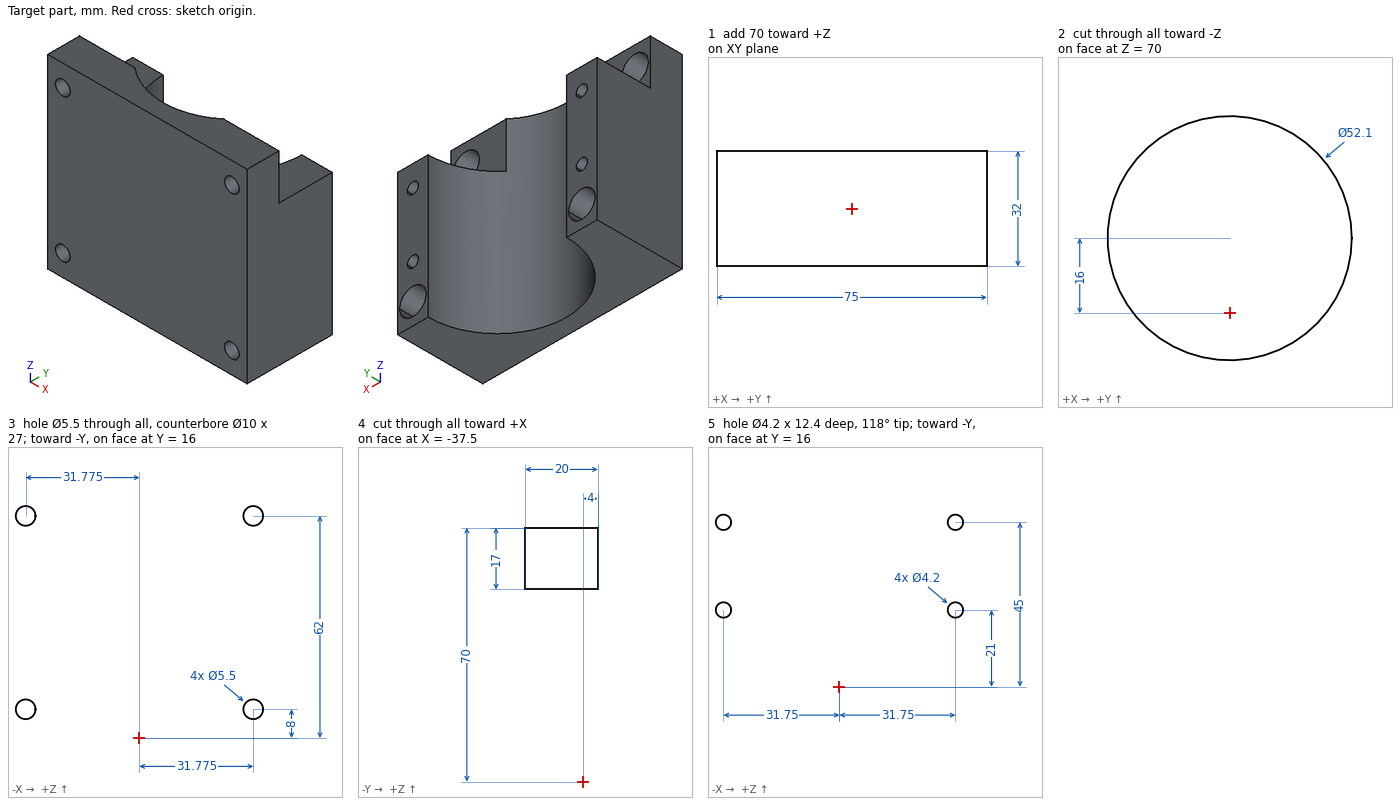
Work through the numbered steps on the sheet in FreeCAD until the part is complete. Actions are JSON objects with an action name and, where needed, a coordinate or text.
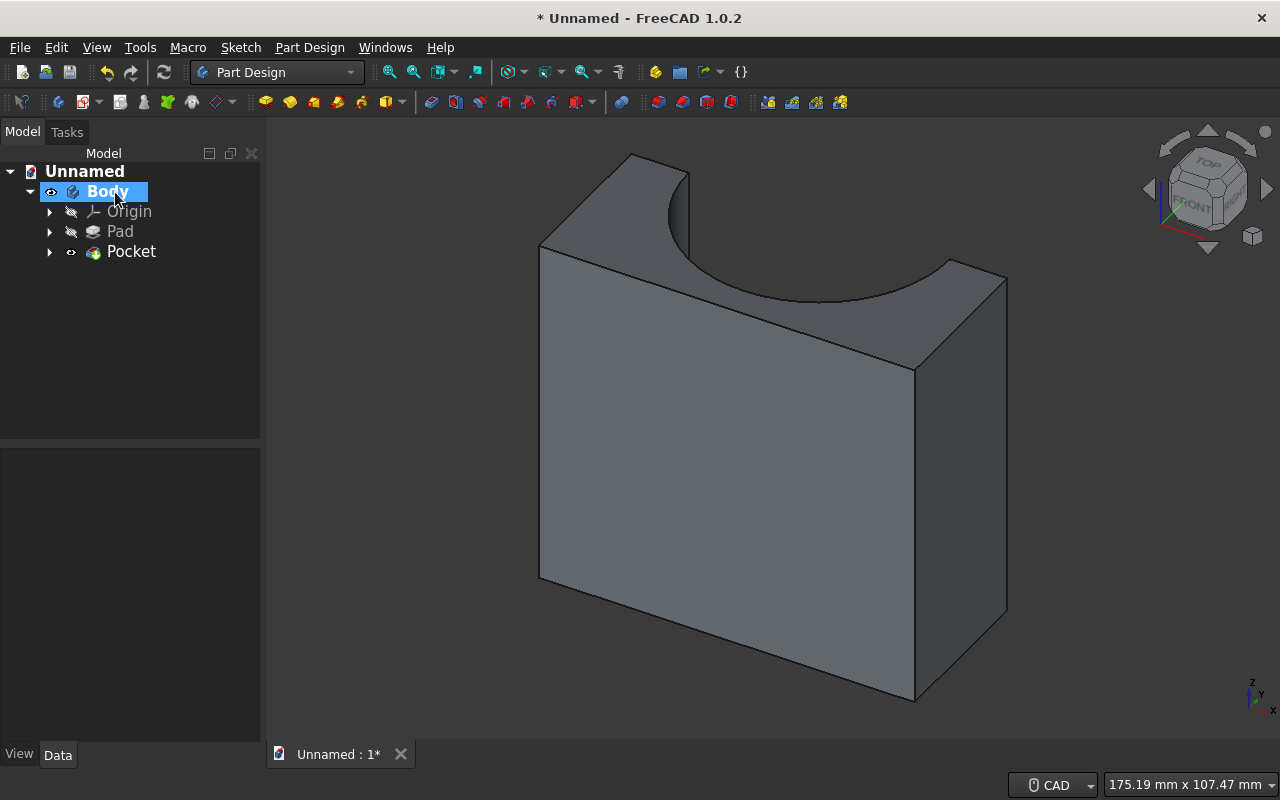
{"action": "key", "text": "4"}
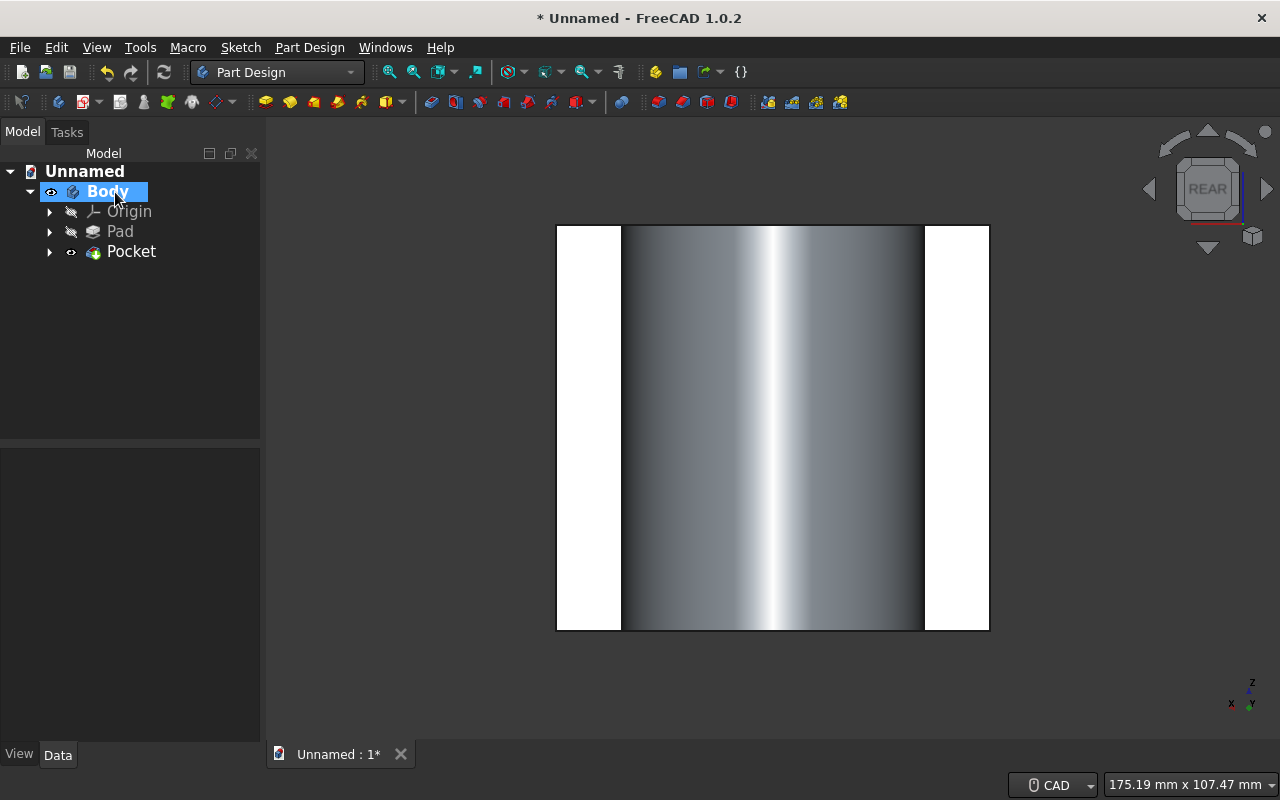
{"action": "left_click", "coordinate": [957, 311]}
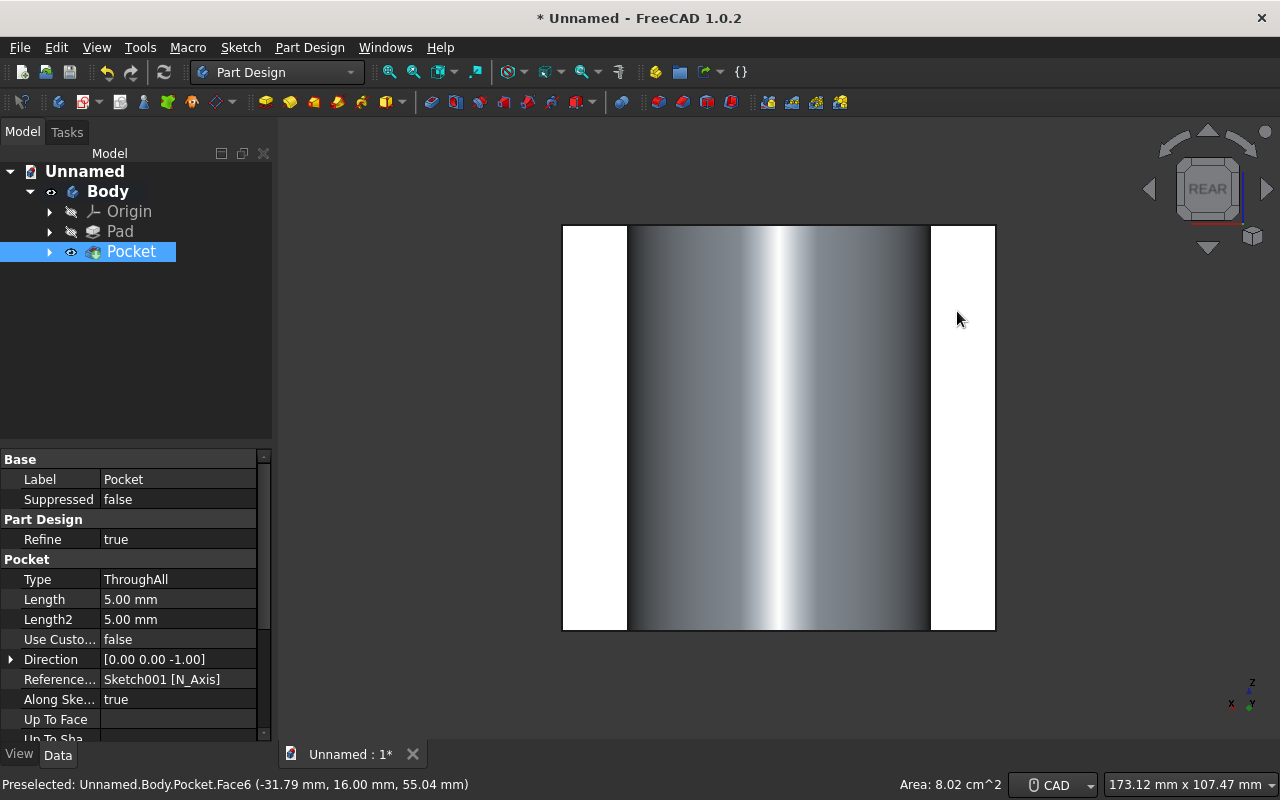
{"action": "left_click", "coordinate": [84, 102]}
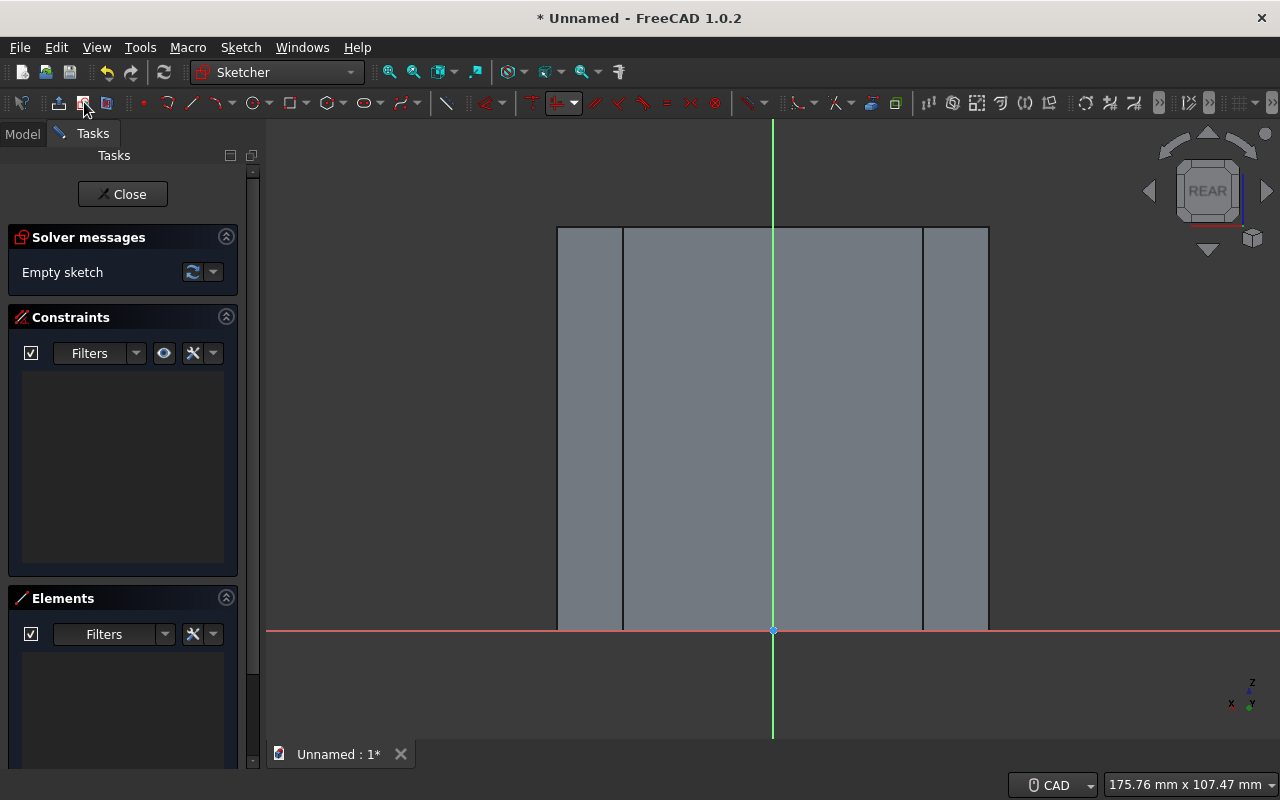
{"action": "left_click", "coordinate": [254, 104]}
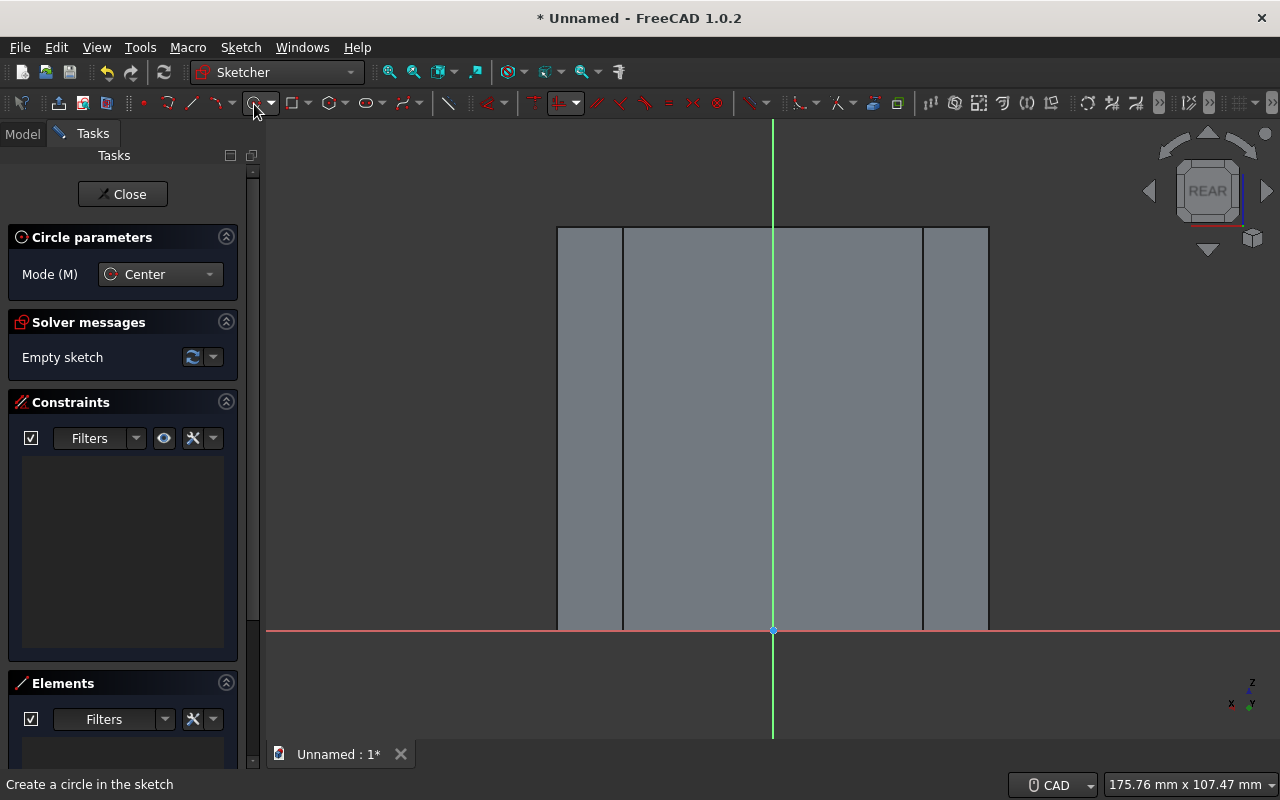
{"action": "scroll", "coordinate": [956, 585], "scroll_direction": "up", "scroll_amount": 2}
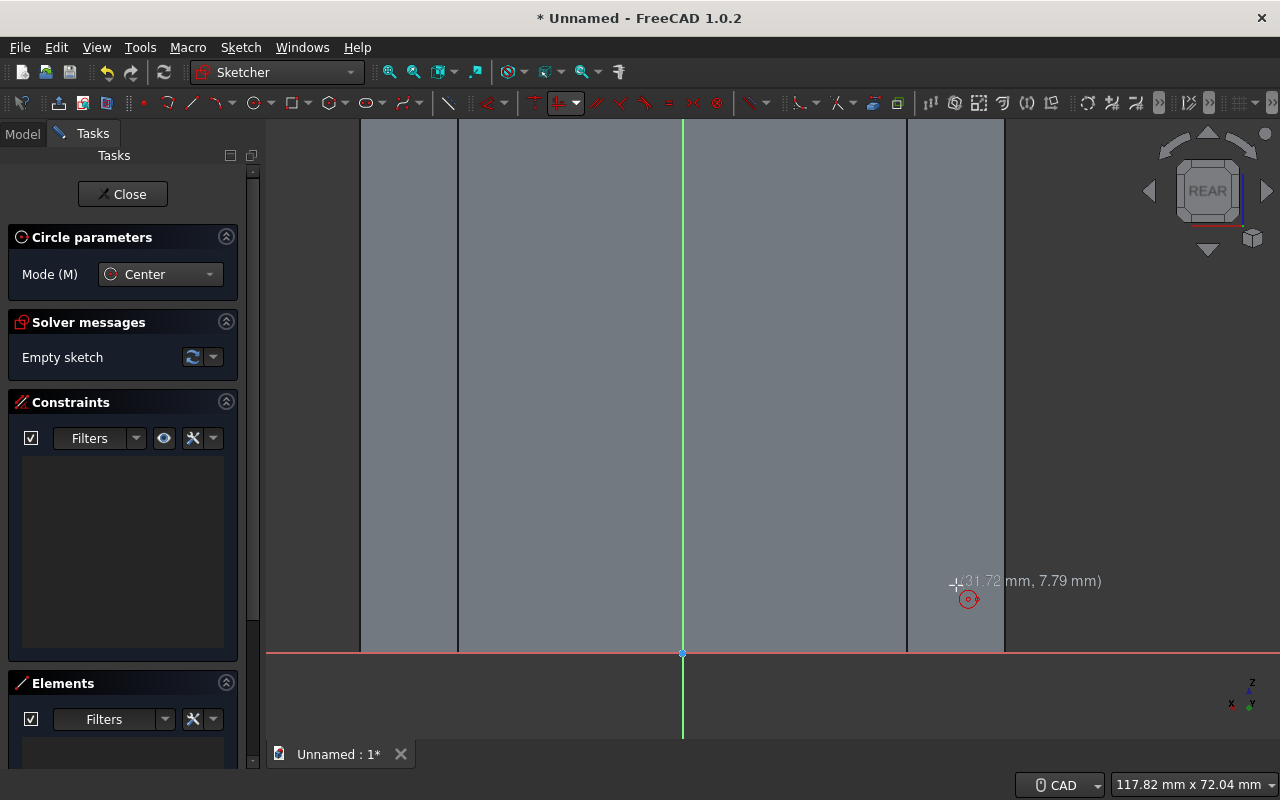
{"action": "left_click", "coordinate": [956, 584]}
{"action": "left_click", "coordinate": [973, 568]}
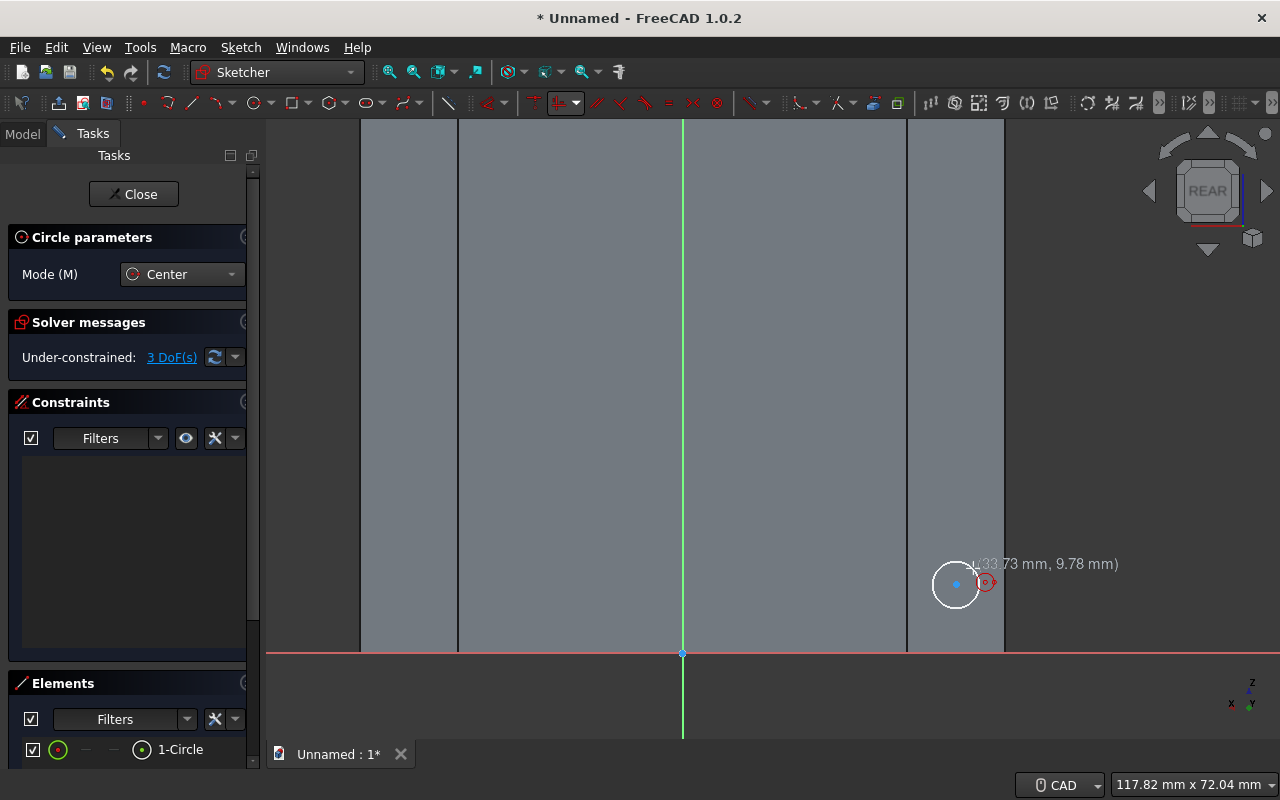
{"action": "scroll", "coordinate": [749, 540], "scroll_direction": "down", "scroll_amount": 2}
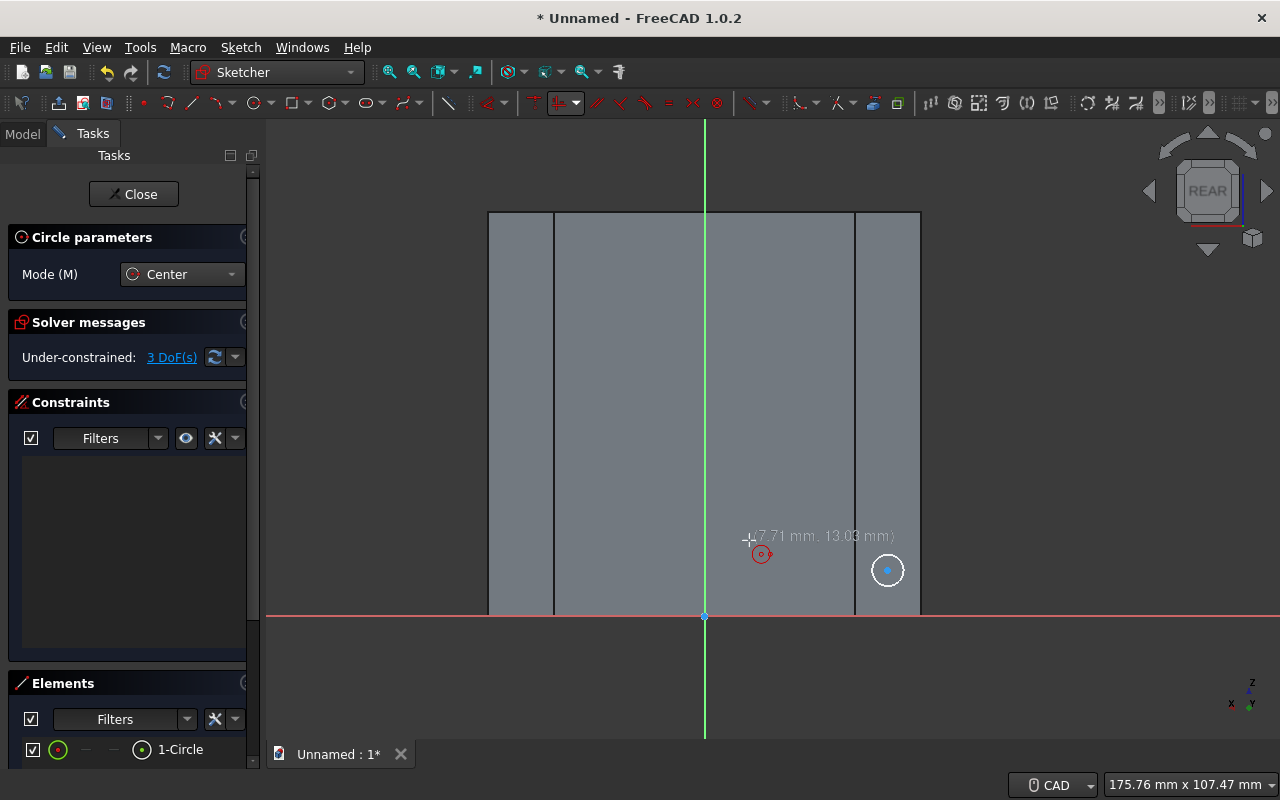
{"action": "scroll", "coordinate": [888, 258], "scroll_direction": "up", "scroll_amount": 2}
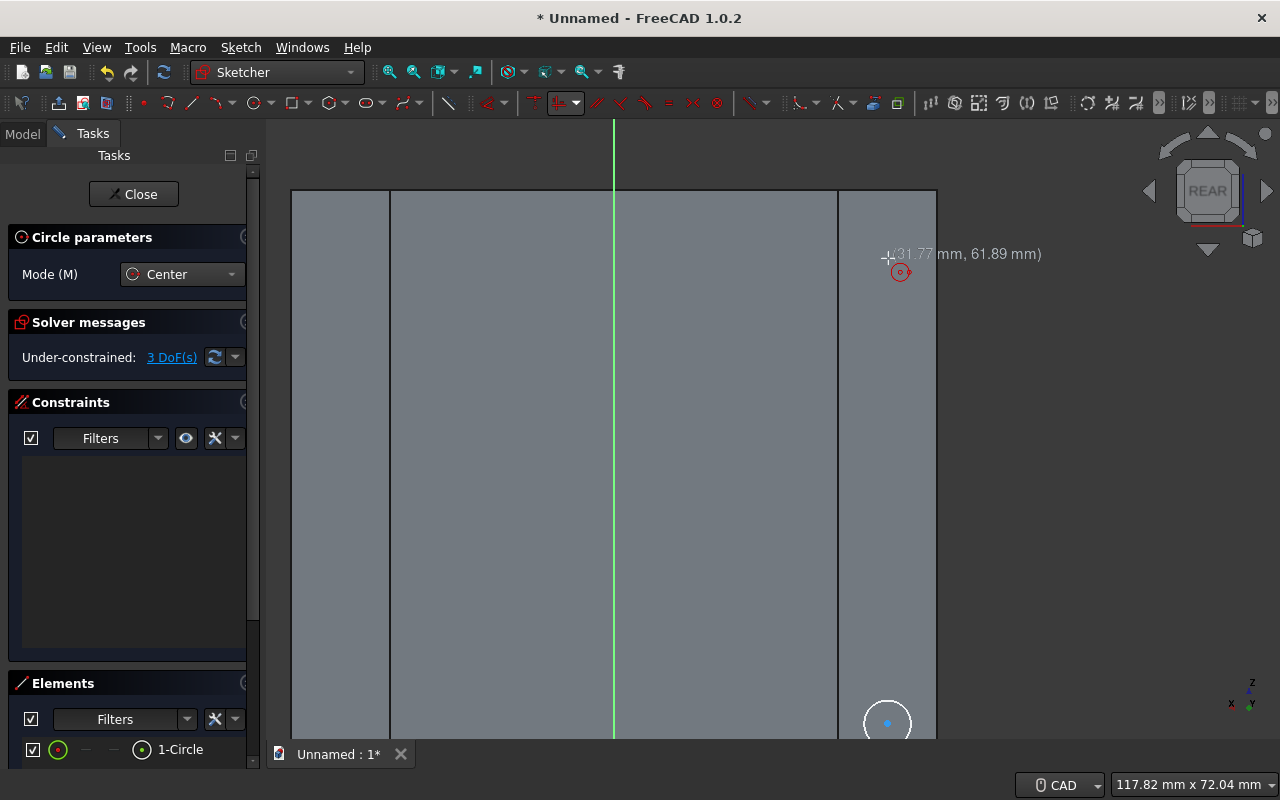
{"action": "left_click", "coordinate": [888, 258]}
{"action": "left_click", "coordinate": [904, 242]}